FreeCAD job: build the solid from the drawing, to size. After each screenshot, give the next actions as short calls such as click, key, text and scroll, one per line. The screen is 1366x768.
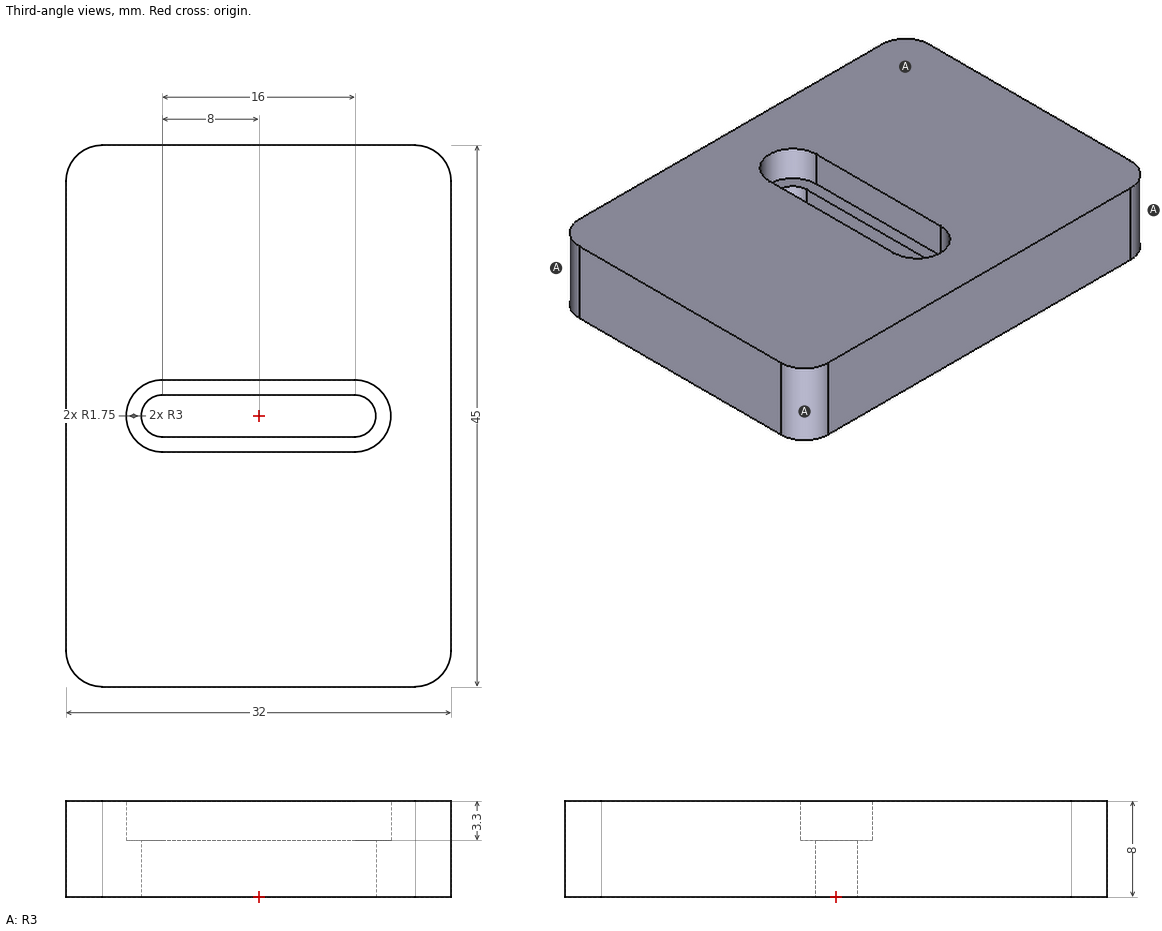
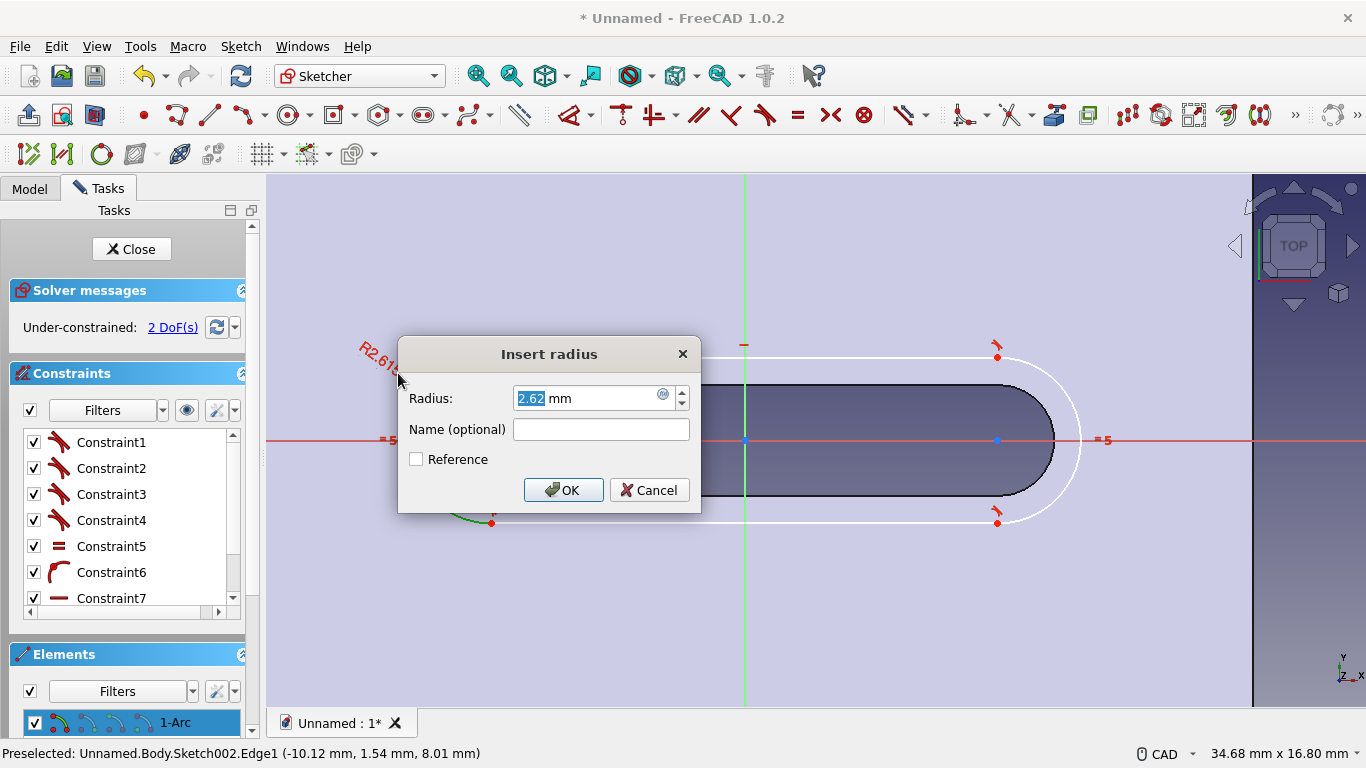
text(3)
key(Return)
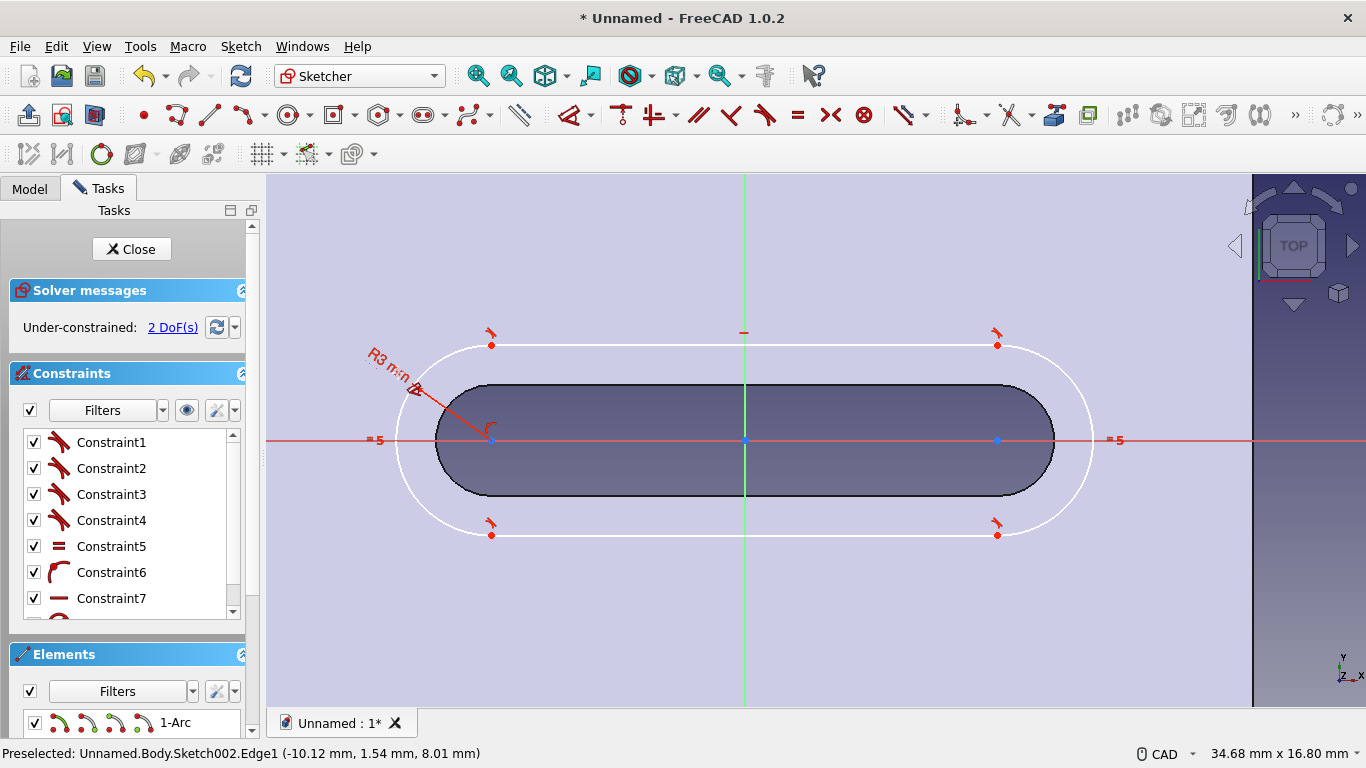
click(643, 345)
click(628, 311)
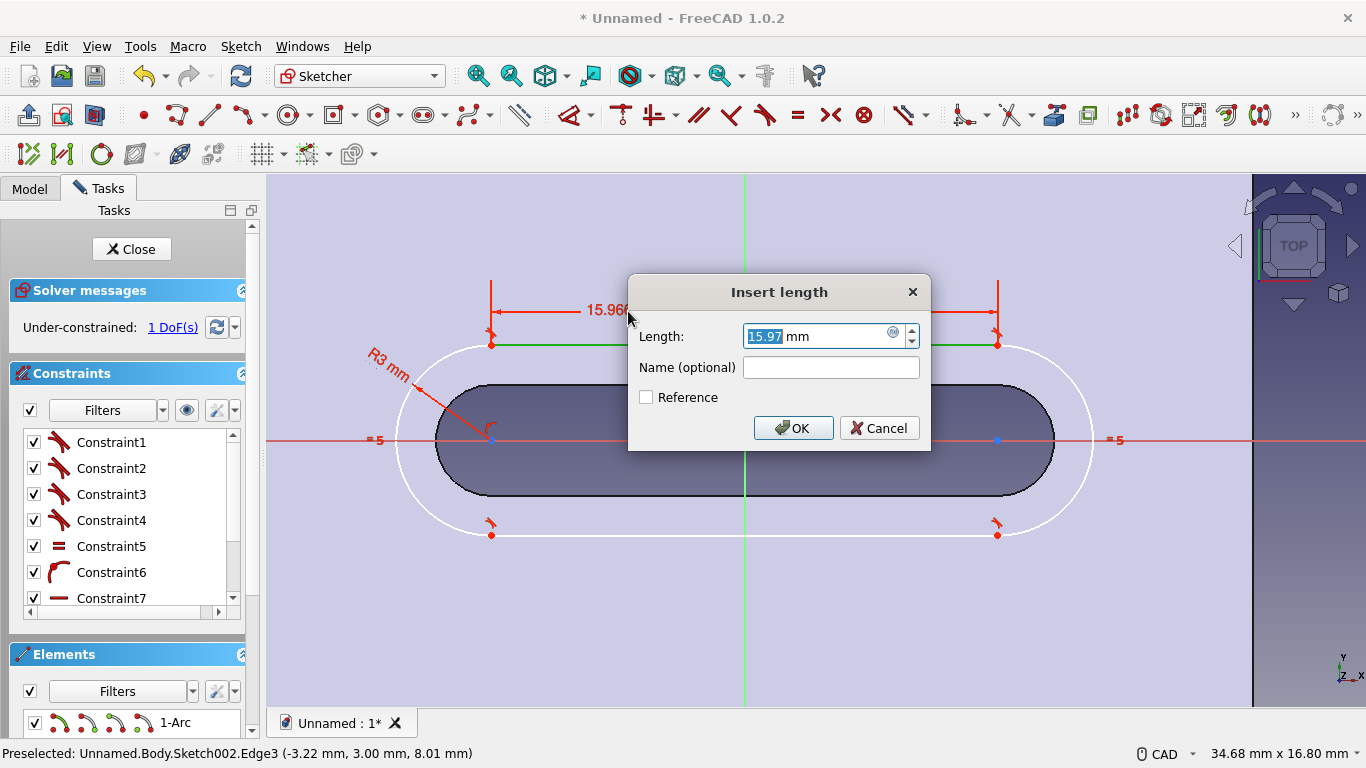
text(16)
key(Return)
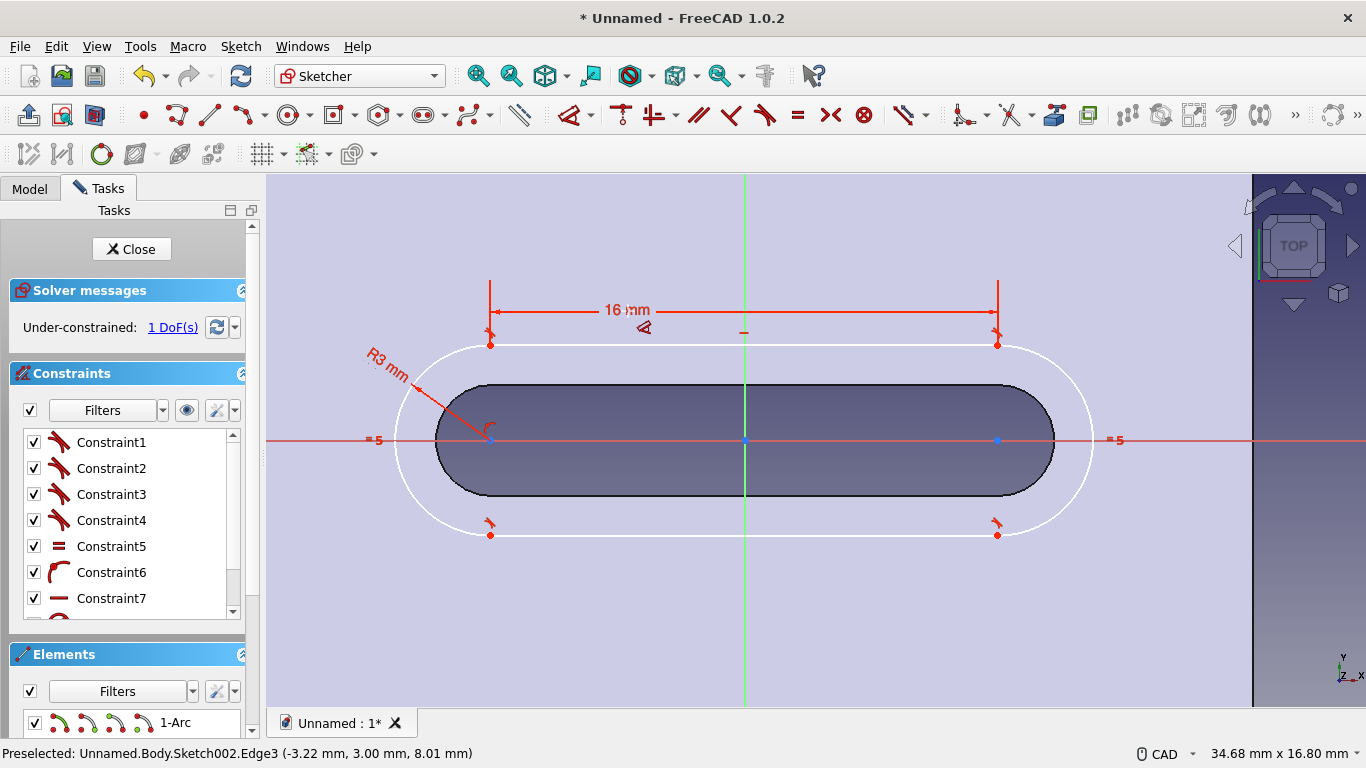
click(490, 345)
click(529, 311)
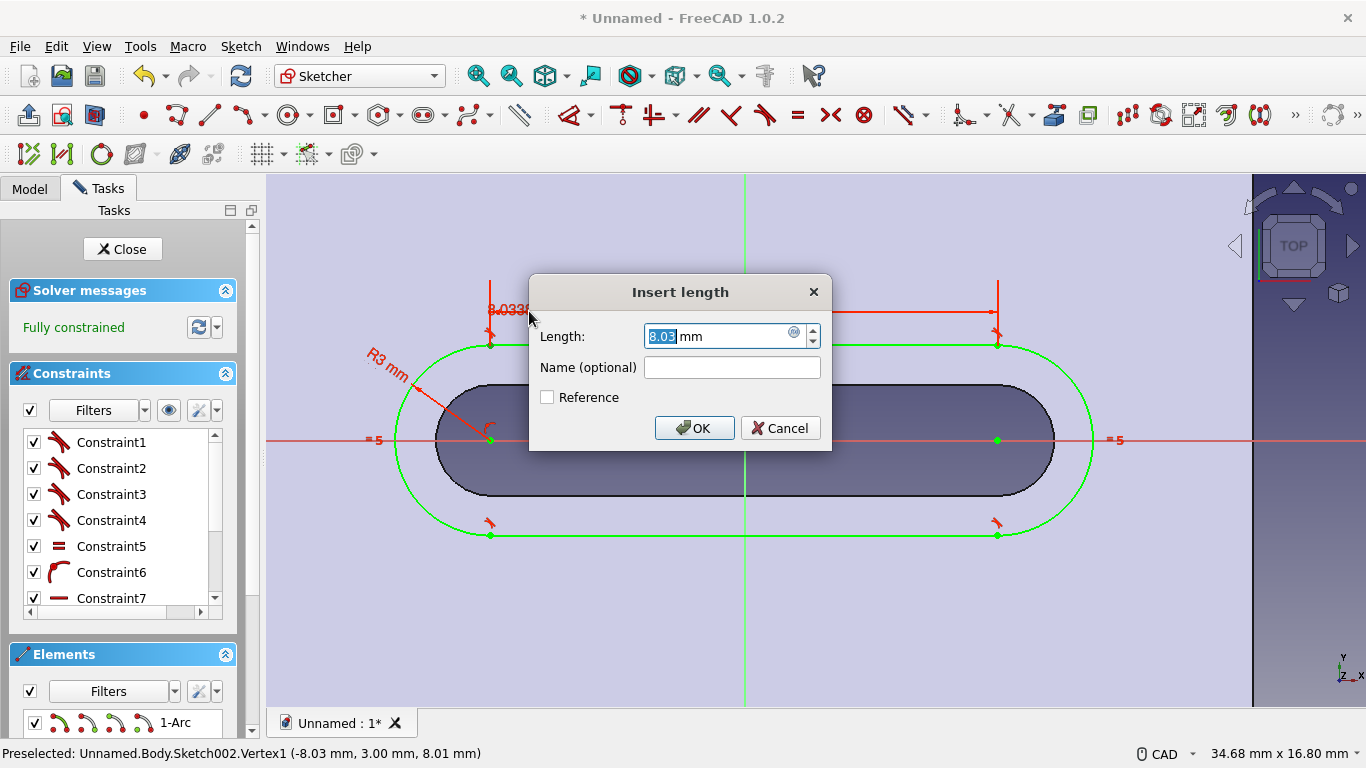
text(8)
key(Return)
key(Escape)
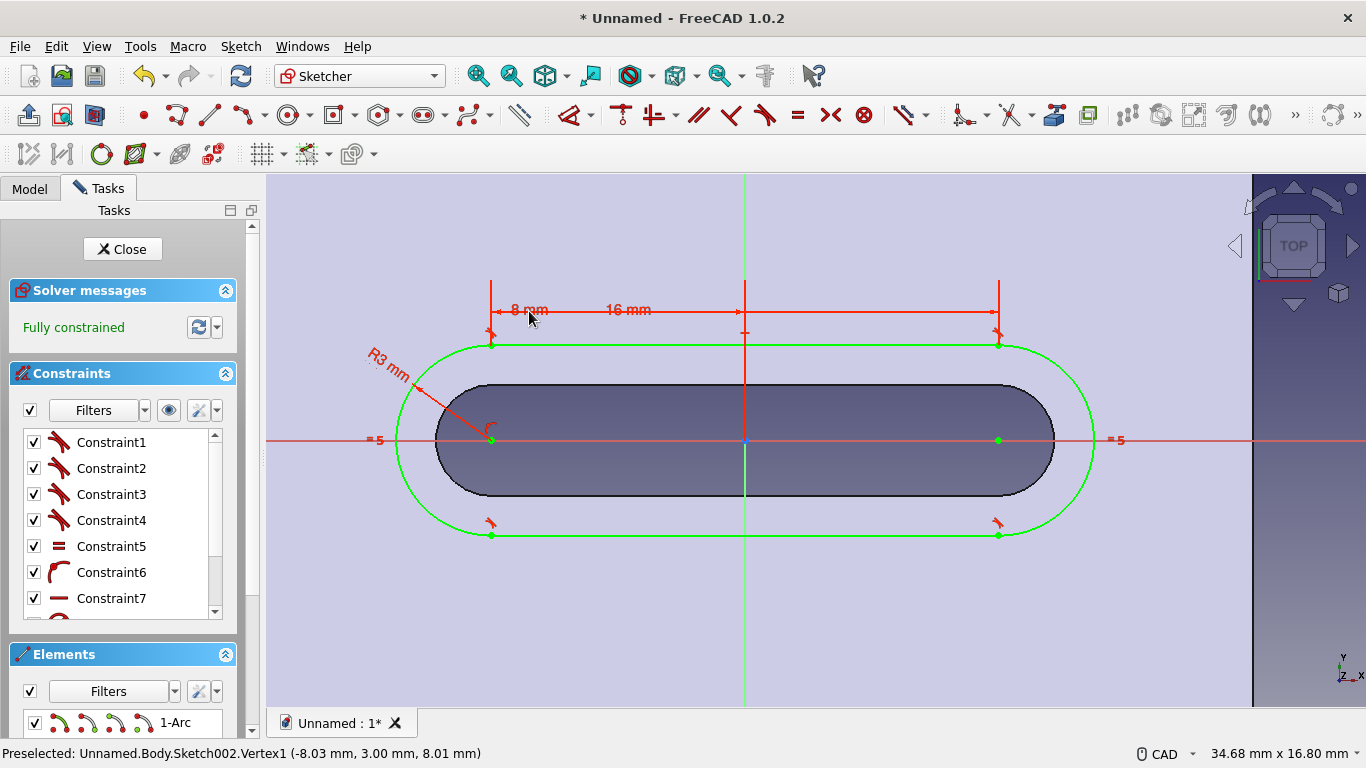
click(123, 249)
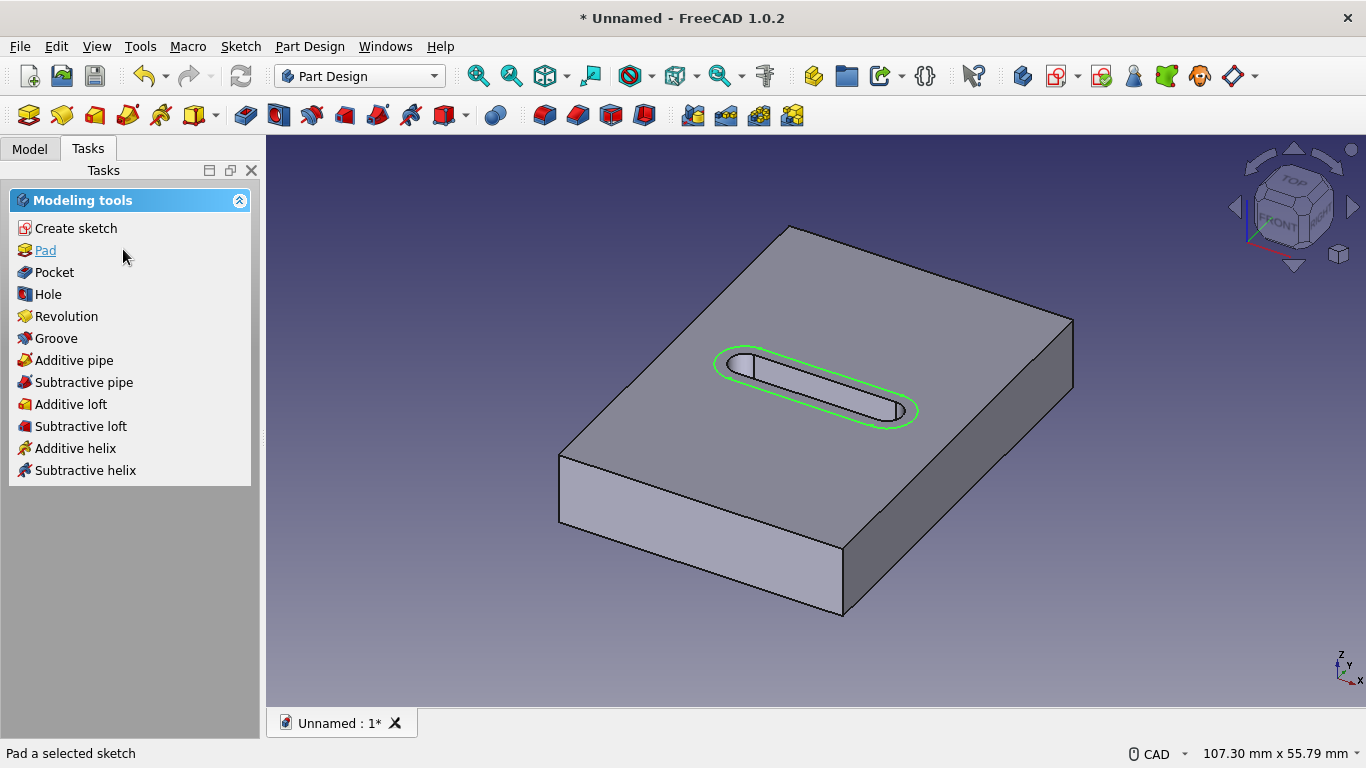
click(246, 116)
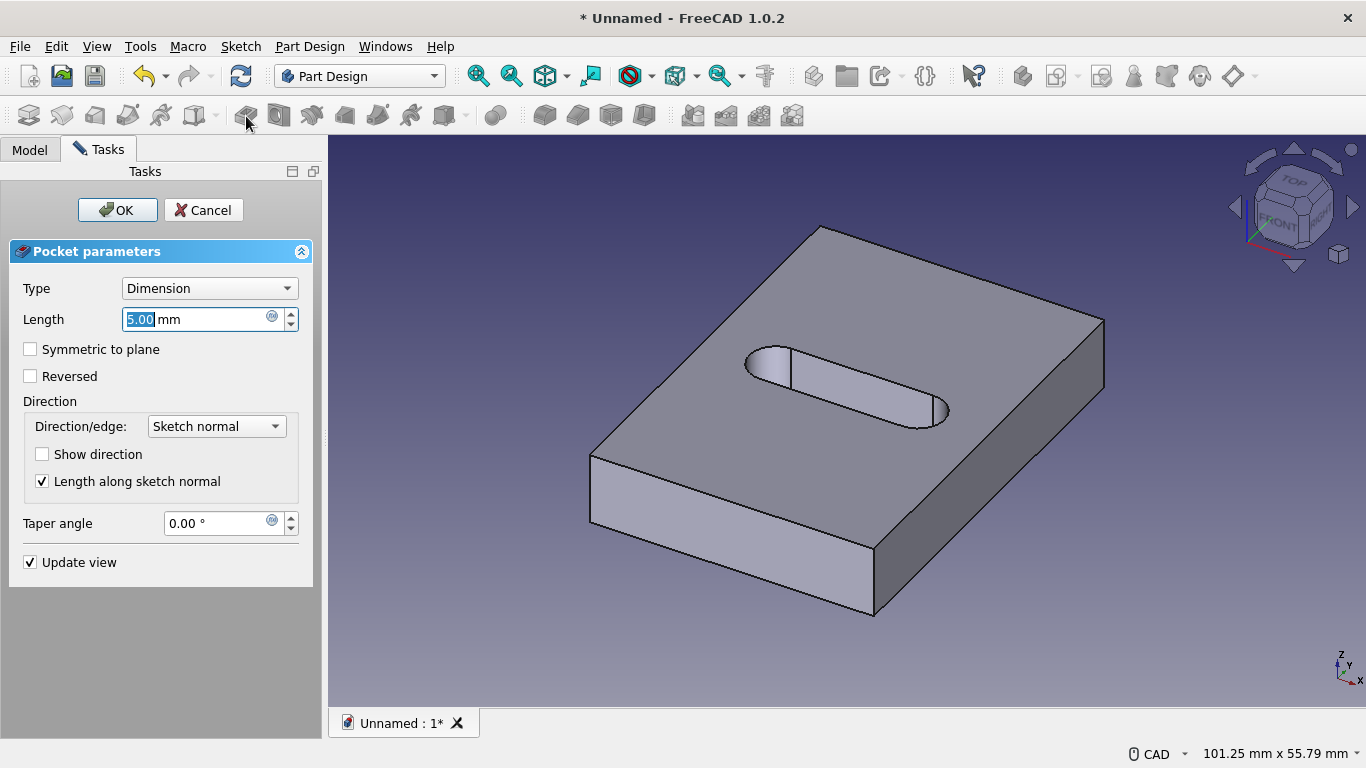
text(3.3)
key(Tab)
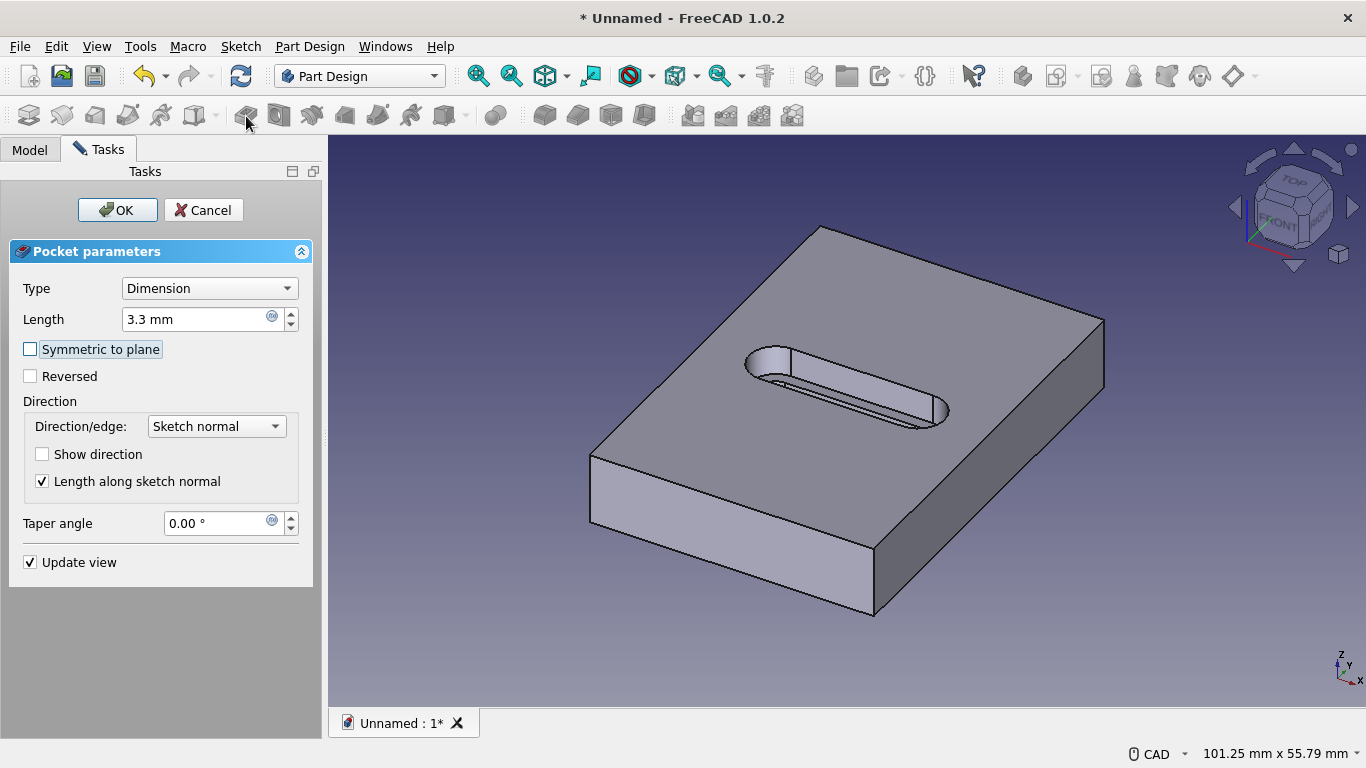
click(118, 210)